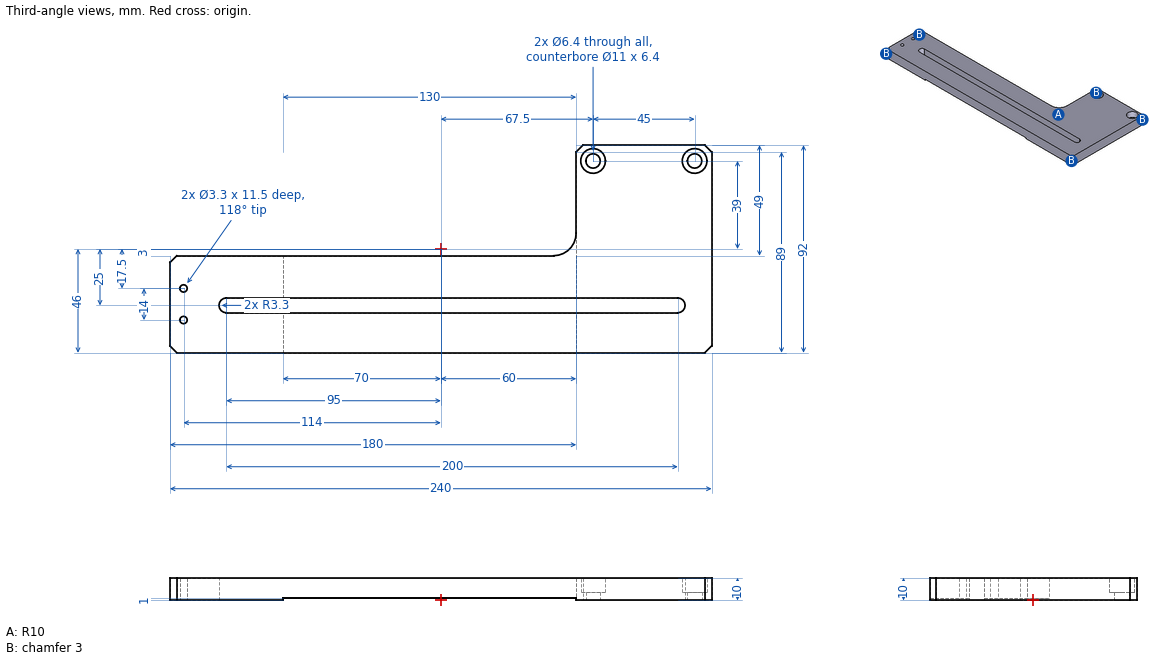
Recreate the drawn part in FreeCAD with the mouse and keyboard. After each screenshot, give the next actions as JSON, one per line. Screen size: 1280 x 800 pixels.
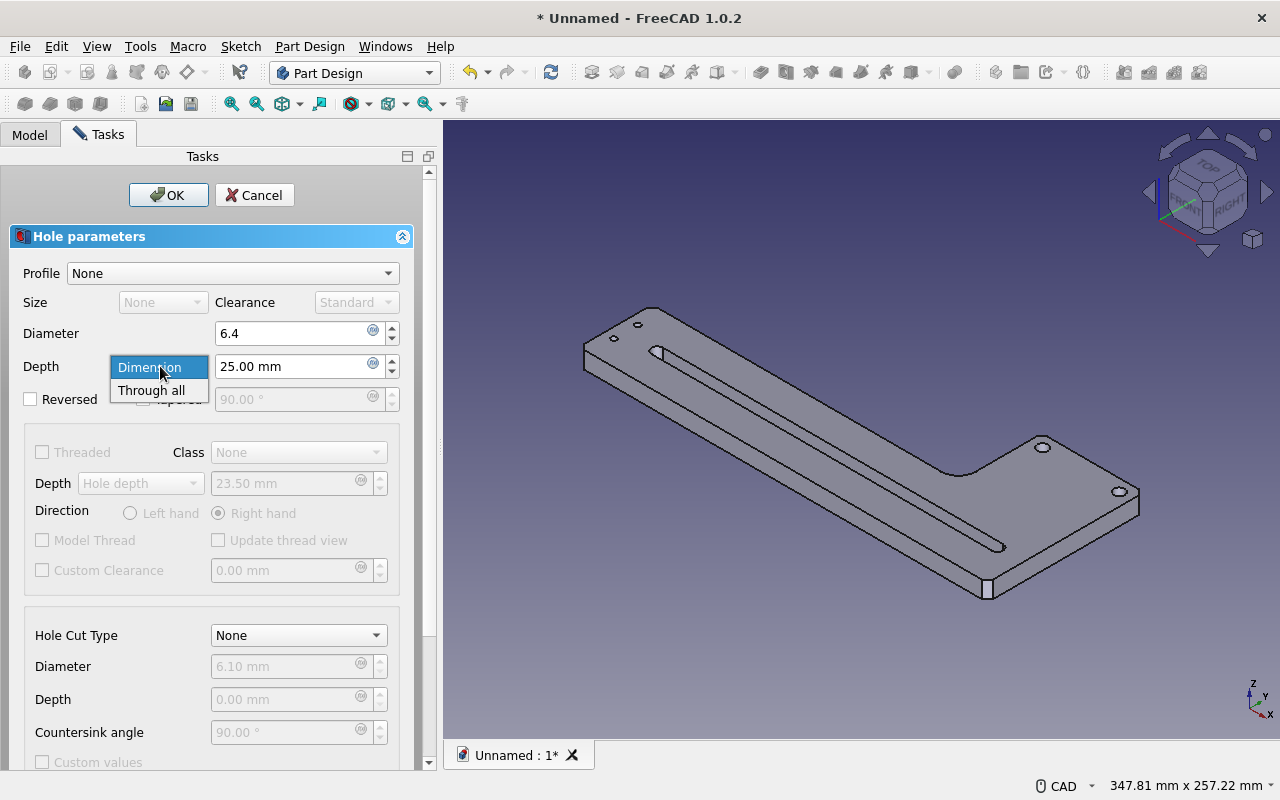
{"action": "left_click", "coordinate": [158, 390]}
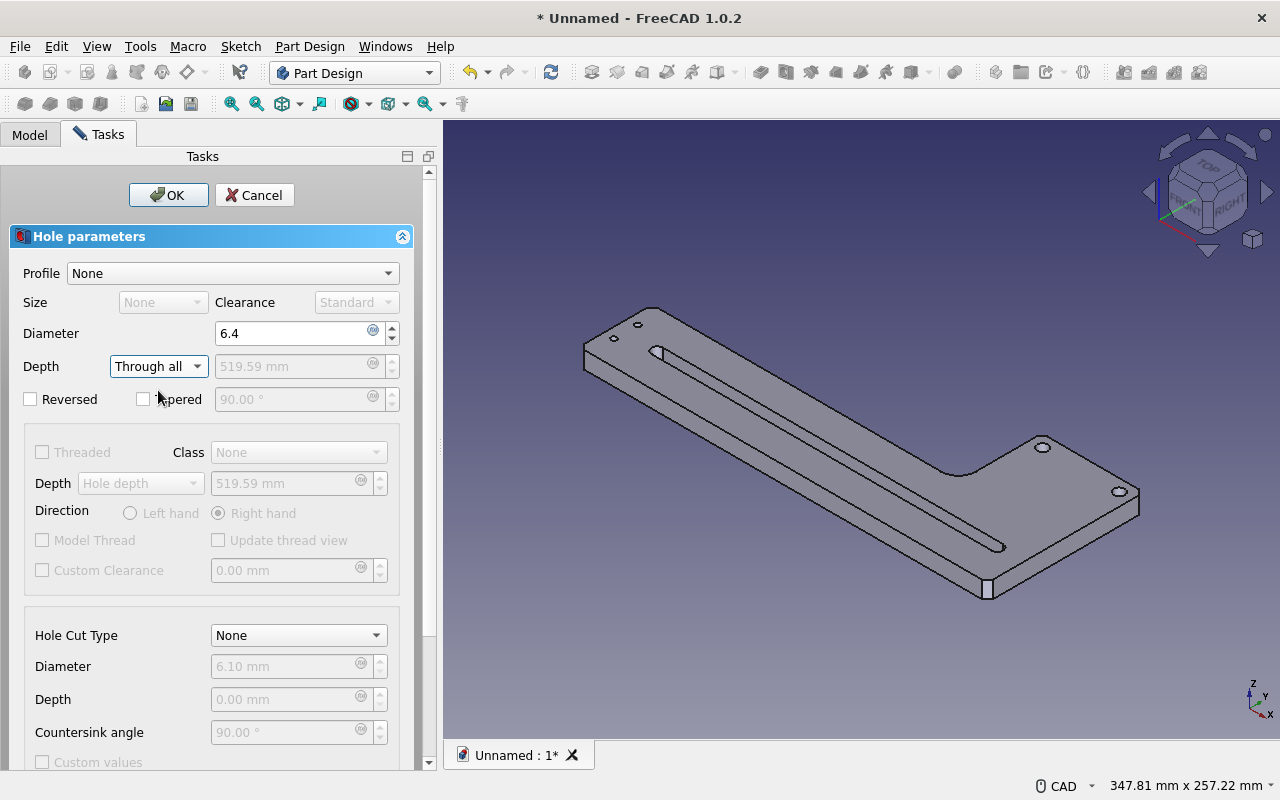
{"action": "left_click", "coordinate": [300, 636]}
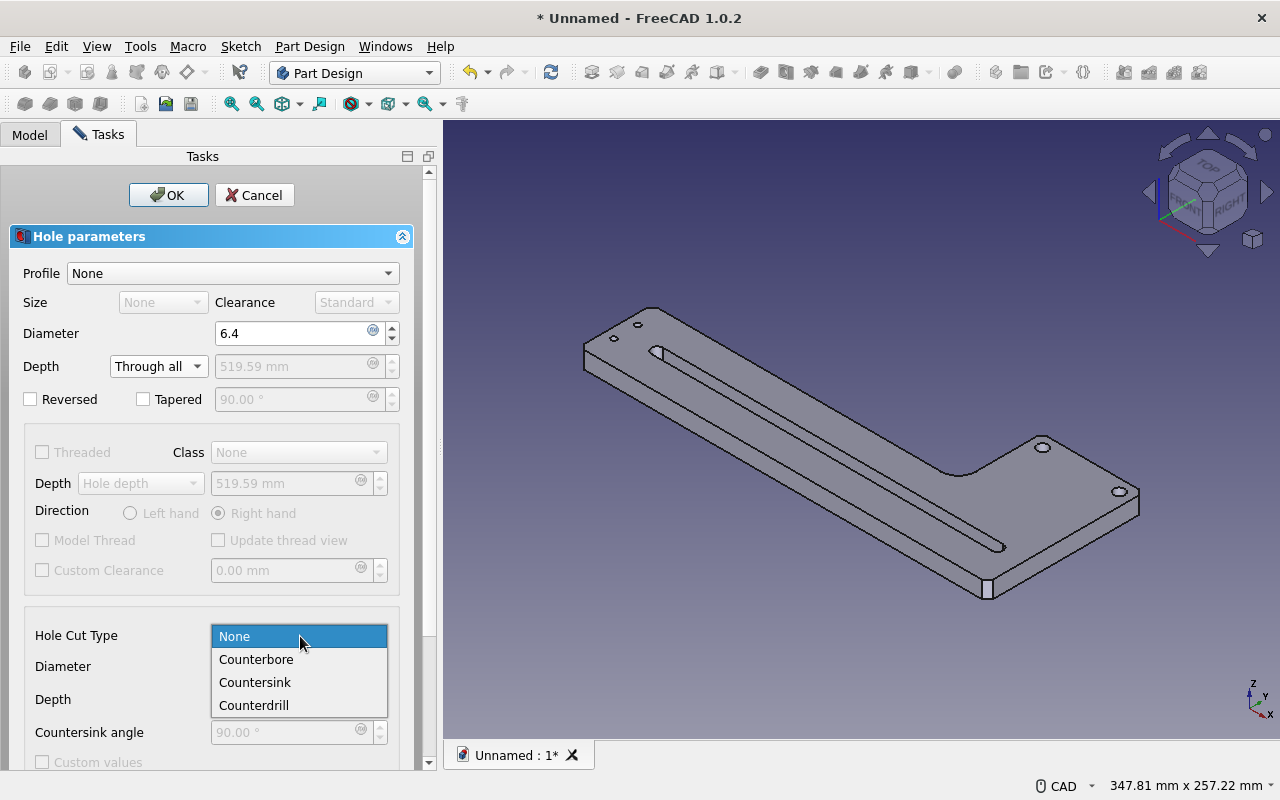
{"action": "left_click", "coordinate": [298, 660]}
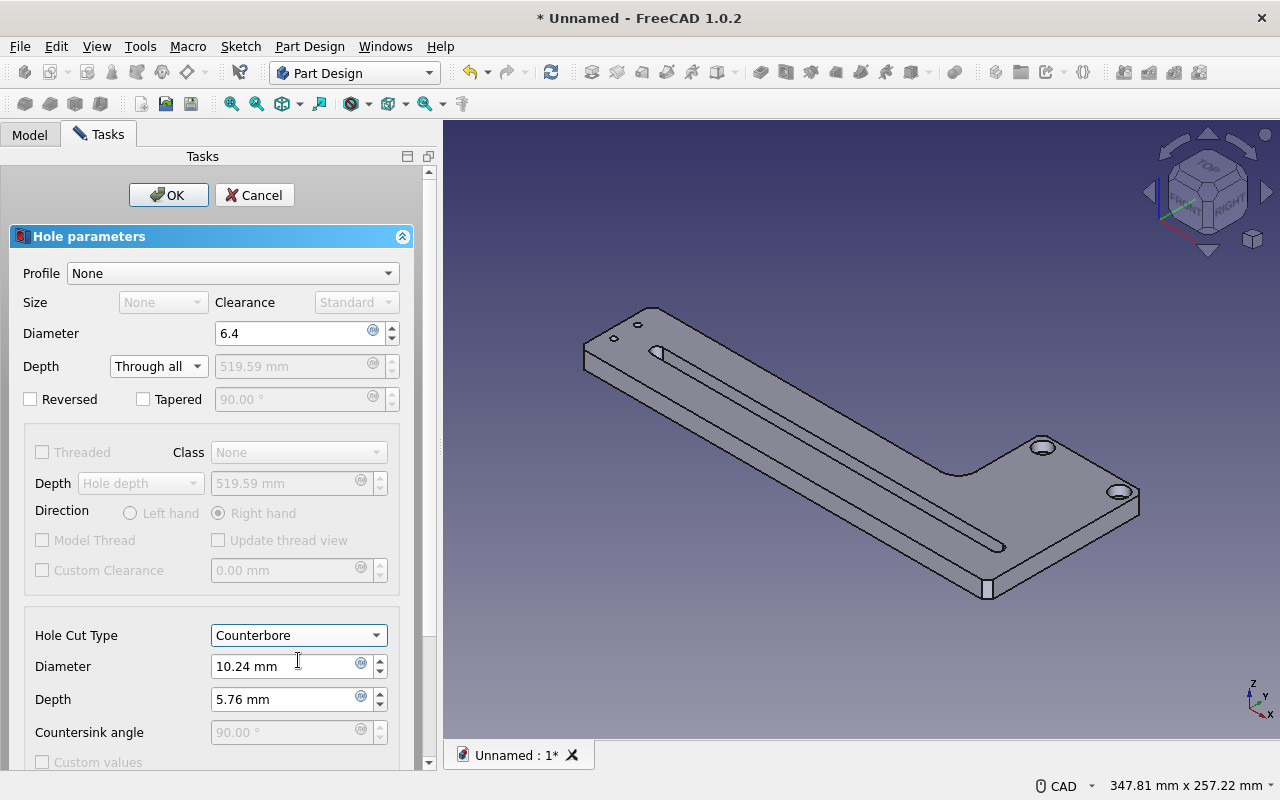
{"action": "triple_click", "coordinate": [292, 666]}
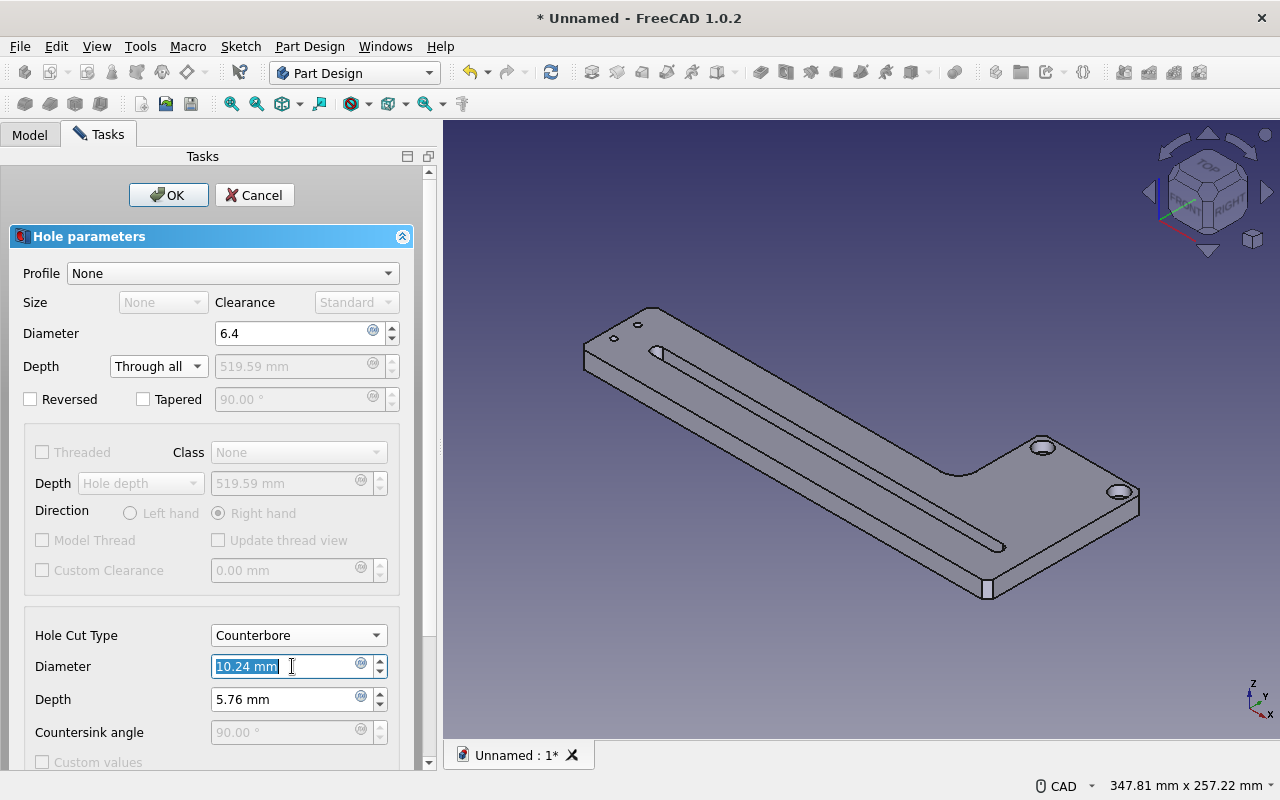
{"action": "type", "text": "11"}
{"action": "key", "text": "Tab"}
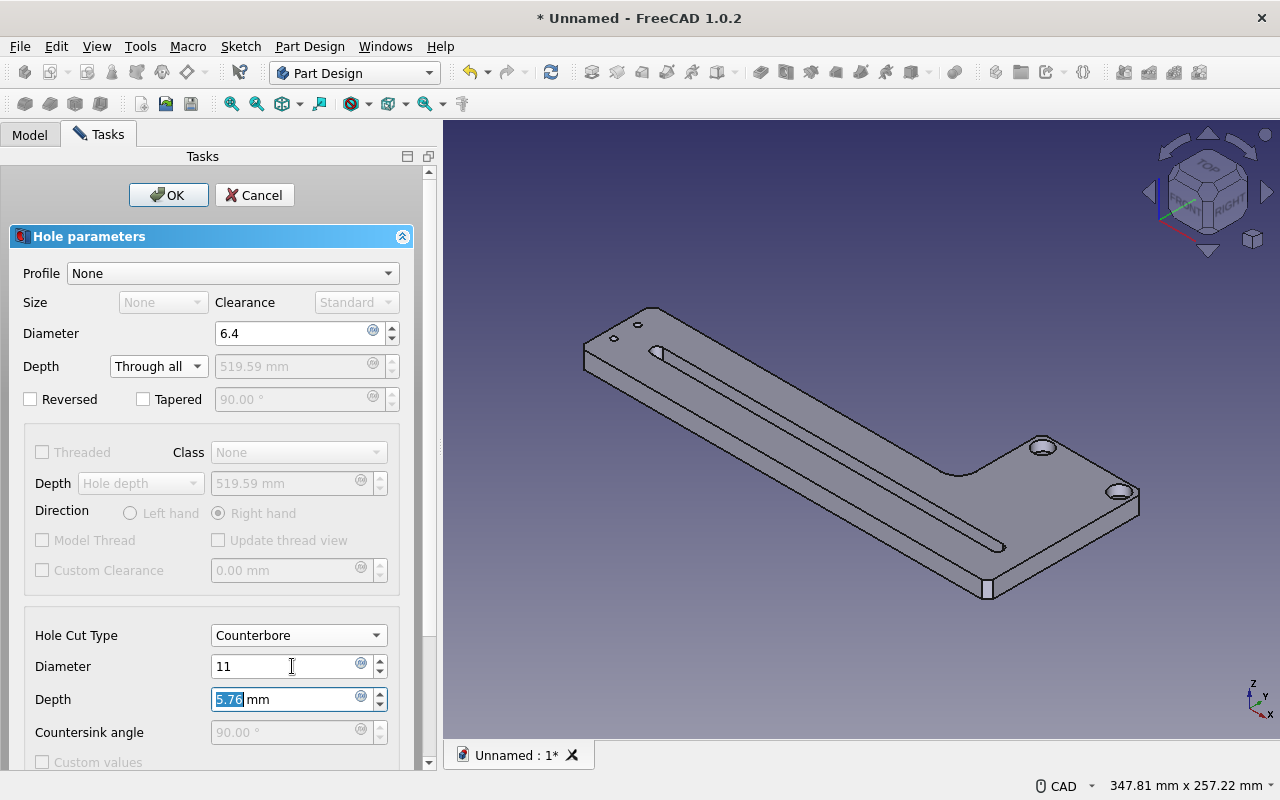
{"action": "type", "text": "6.4"}
{"action": "key", "text": "Tab"}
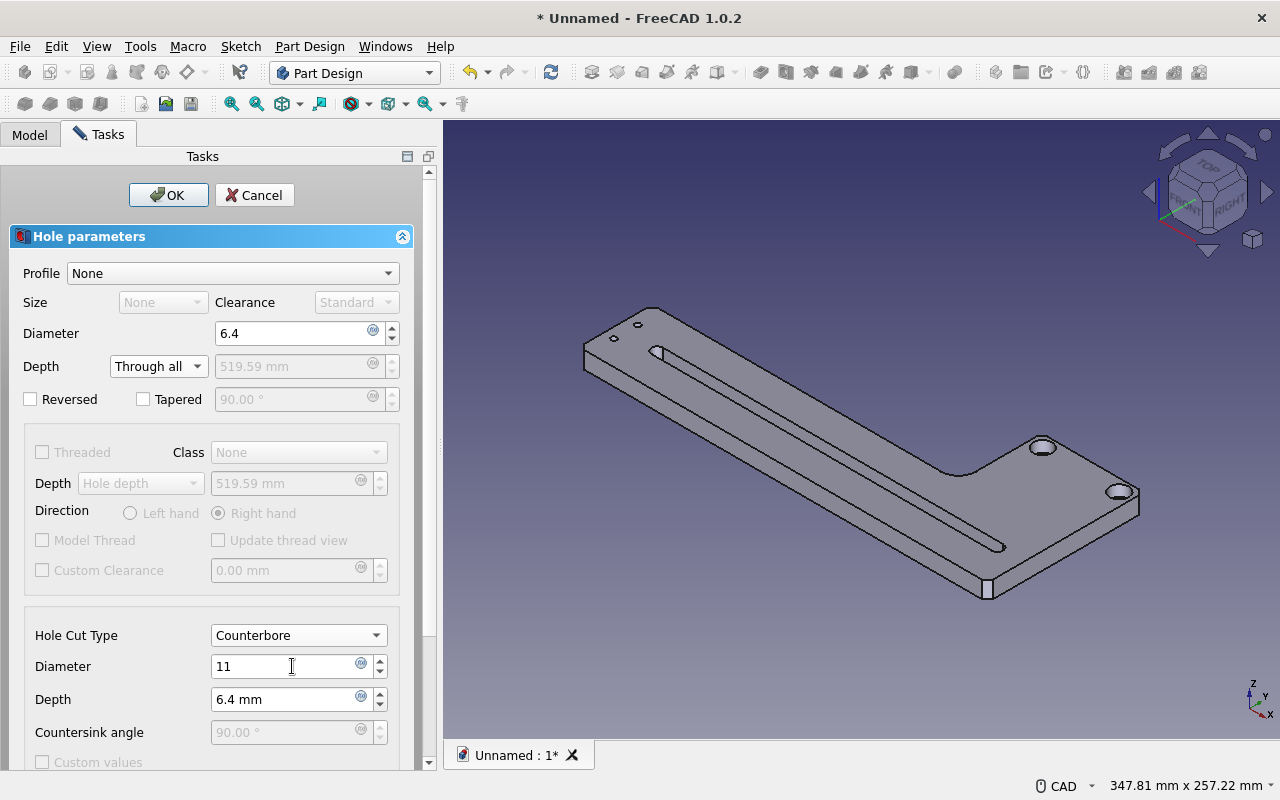
{"action": "left_click", "coordinate": [169, 195]}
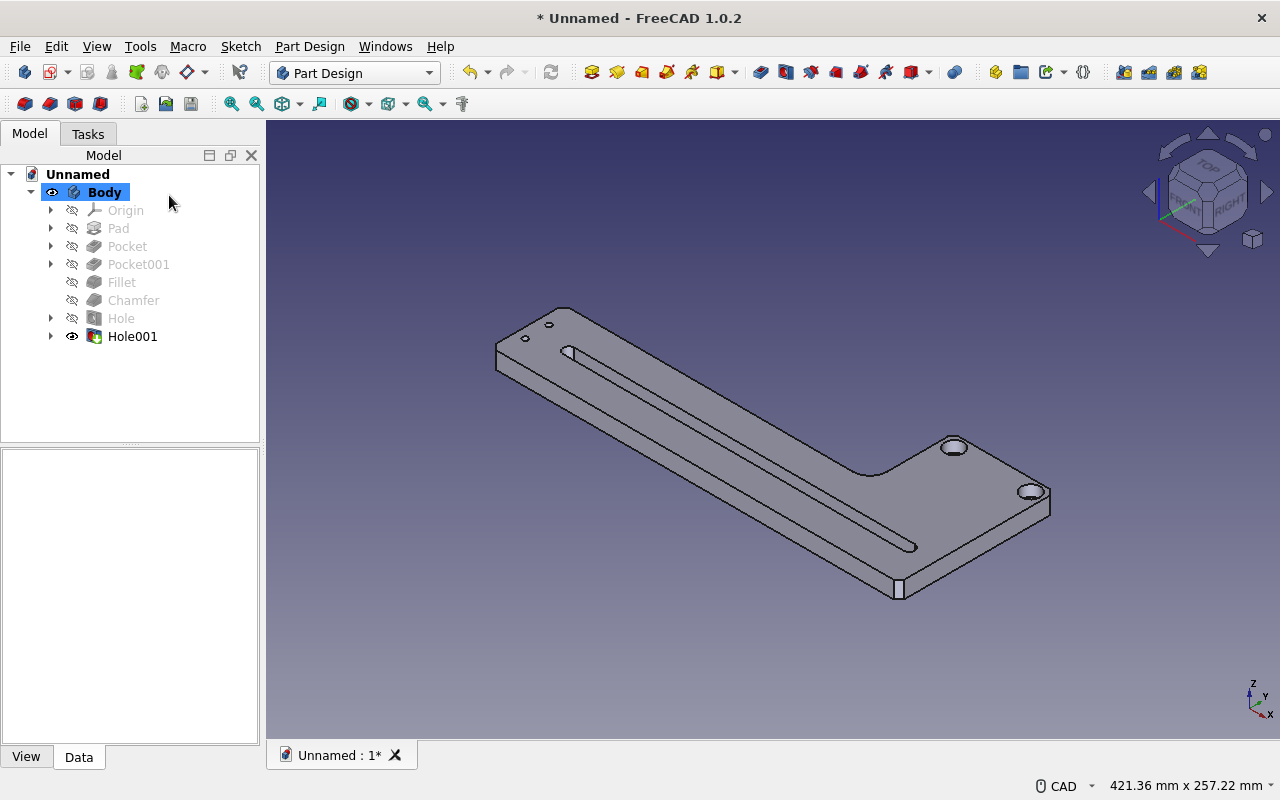
{"action": "key", "text": "5"}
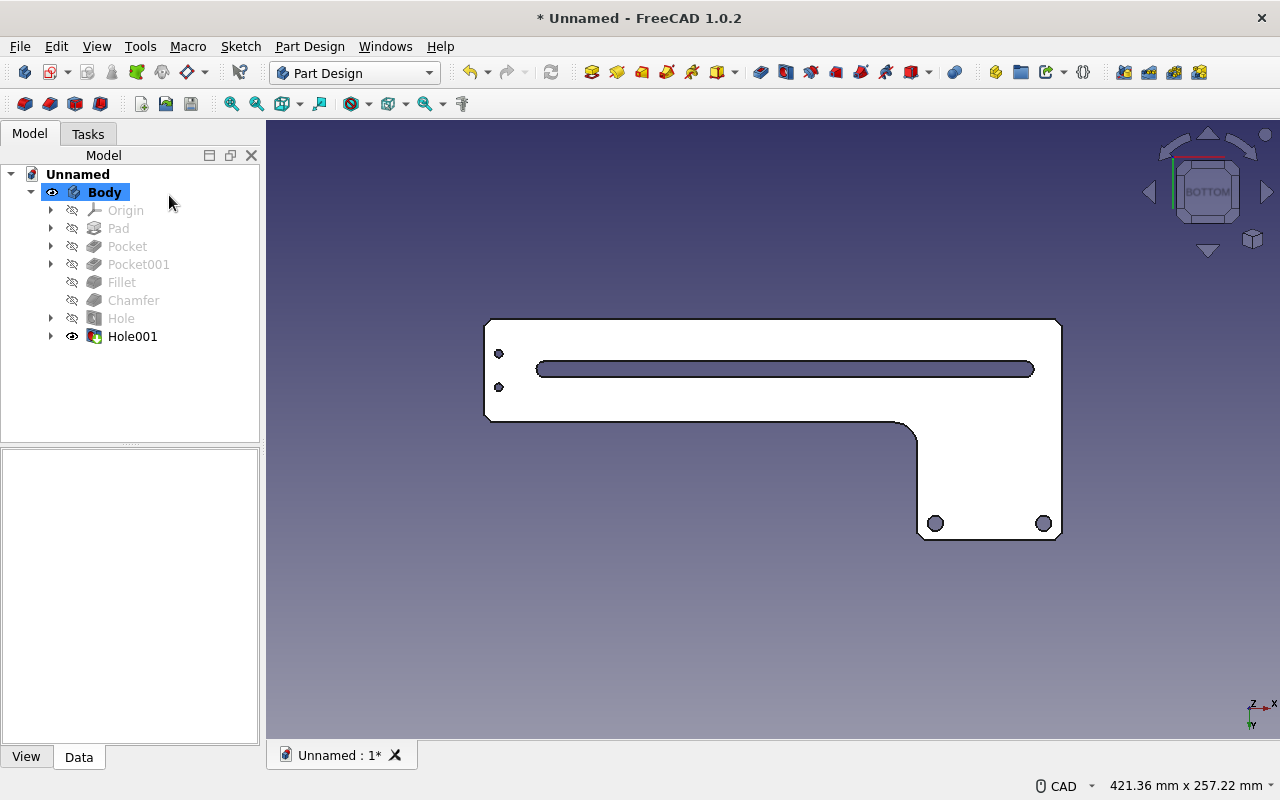
{"action": "left_click", "coordinate": [1021, 460]}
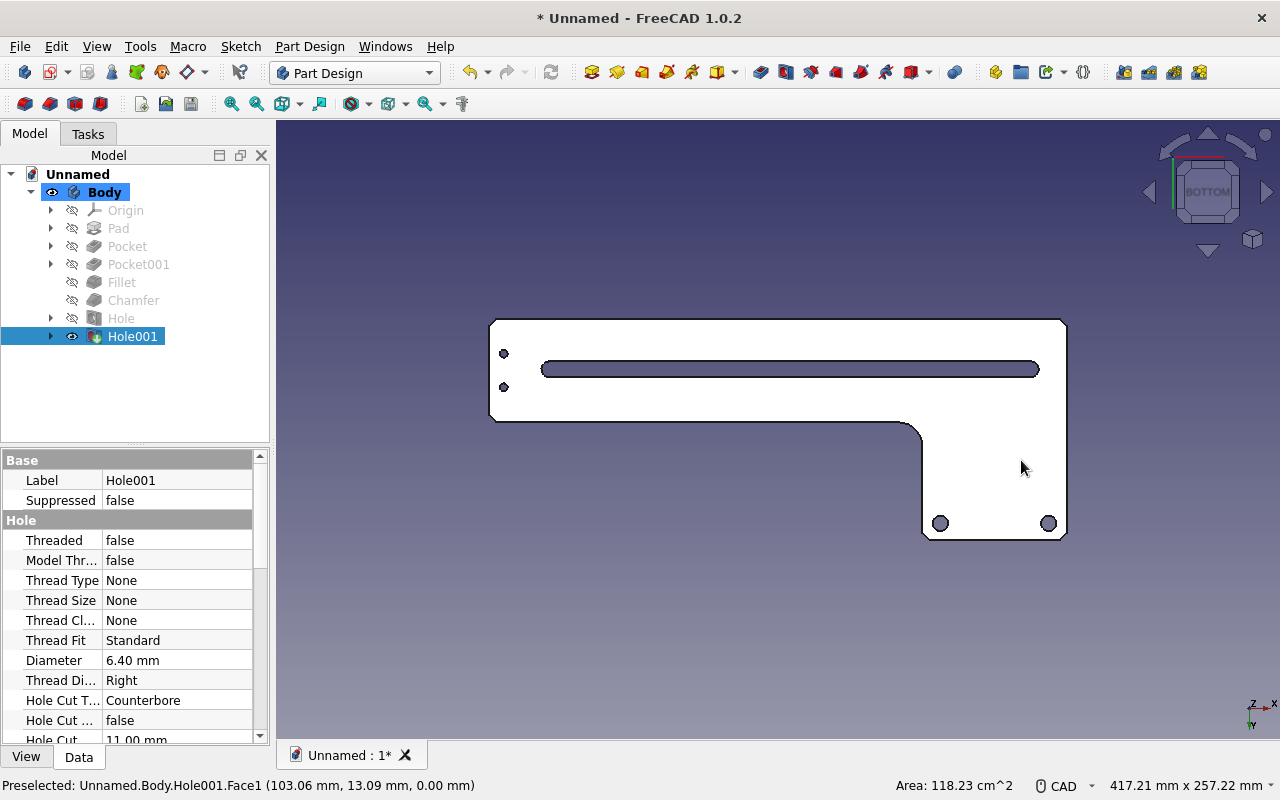
{"action": "left_click", "coordinate": [50, 72]}